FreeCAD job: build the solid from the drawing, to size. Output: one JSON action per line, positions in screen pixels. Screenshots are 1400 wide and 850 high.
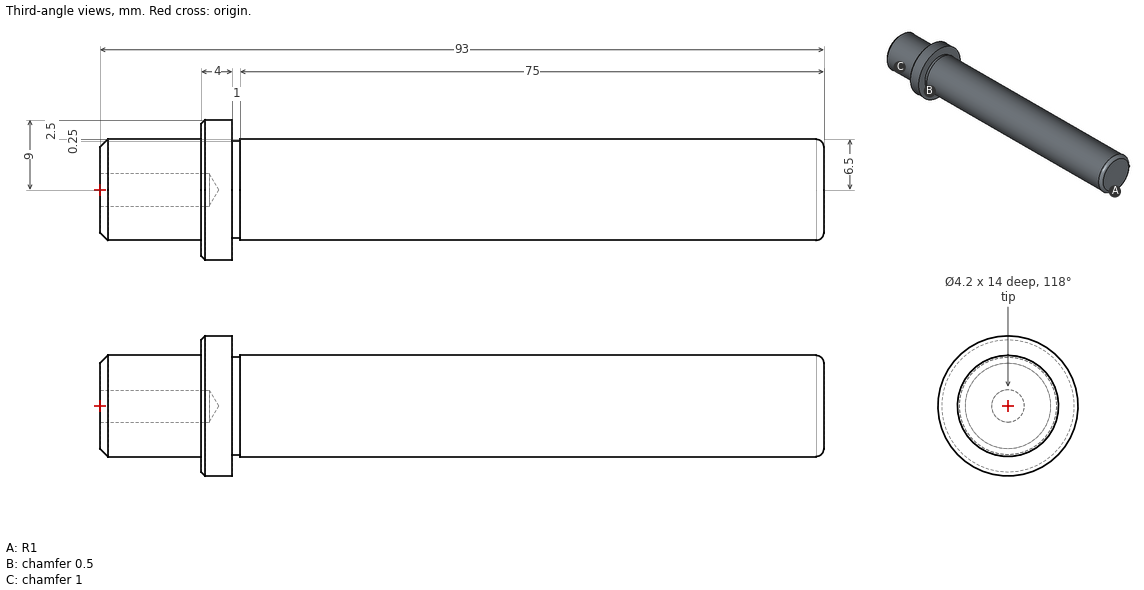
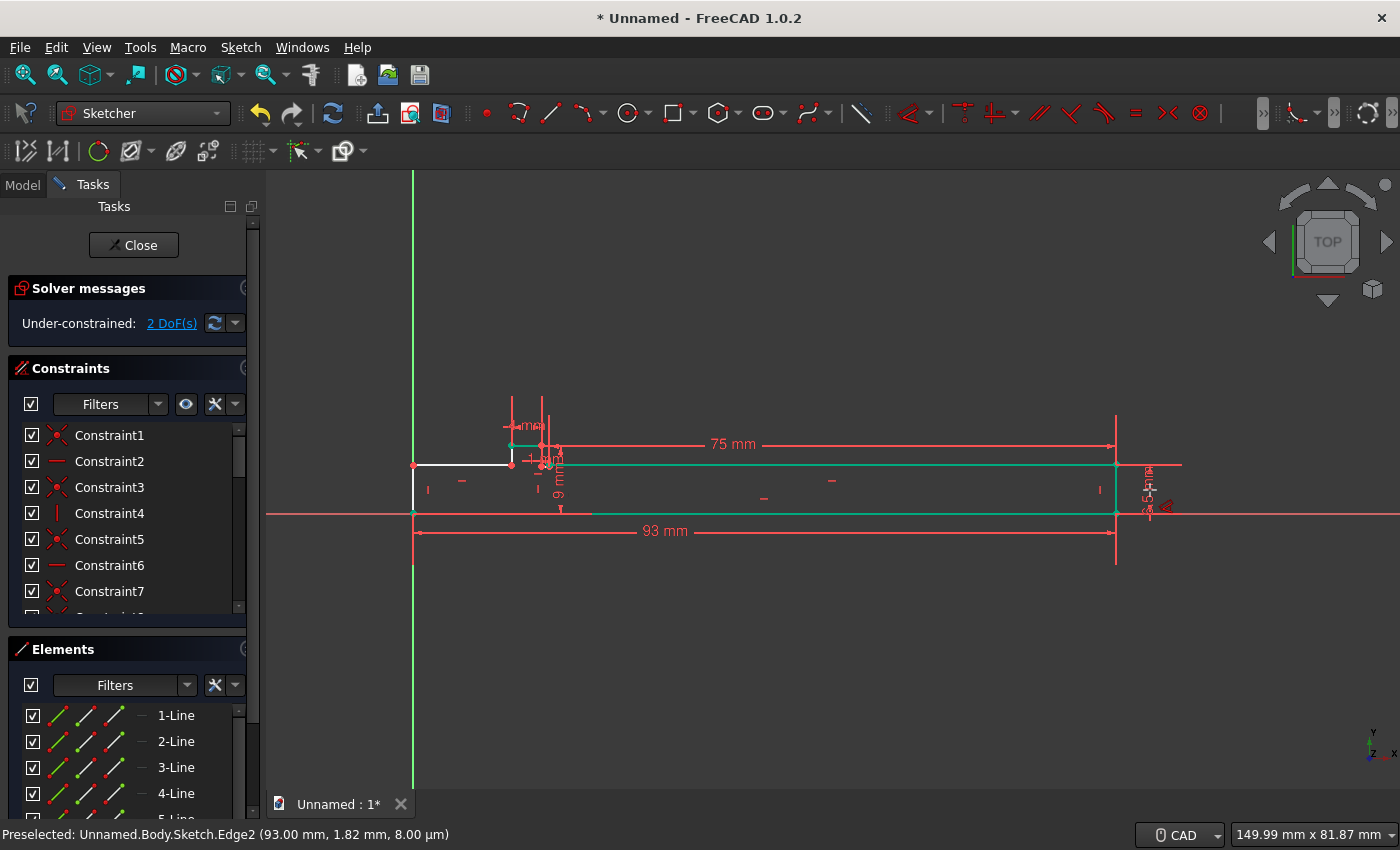
{"action": "scroll", "coordinate": [512, 455], "scroll_direction": "up", "scroll_amount": 4}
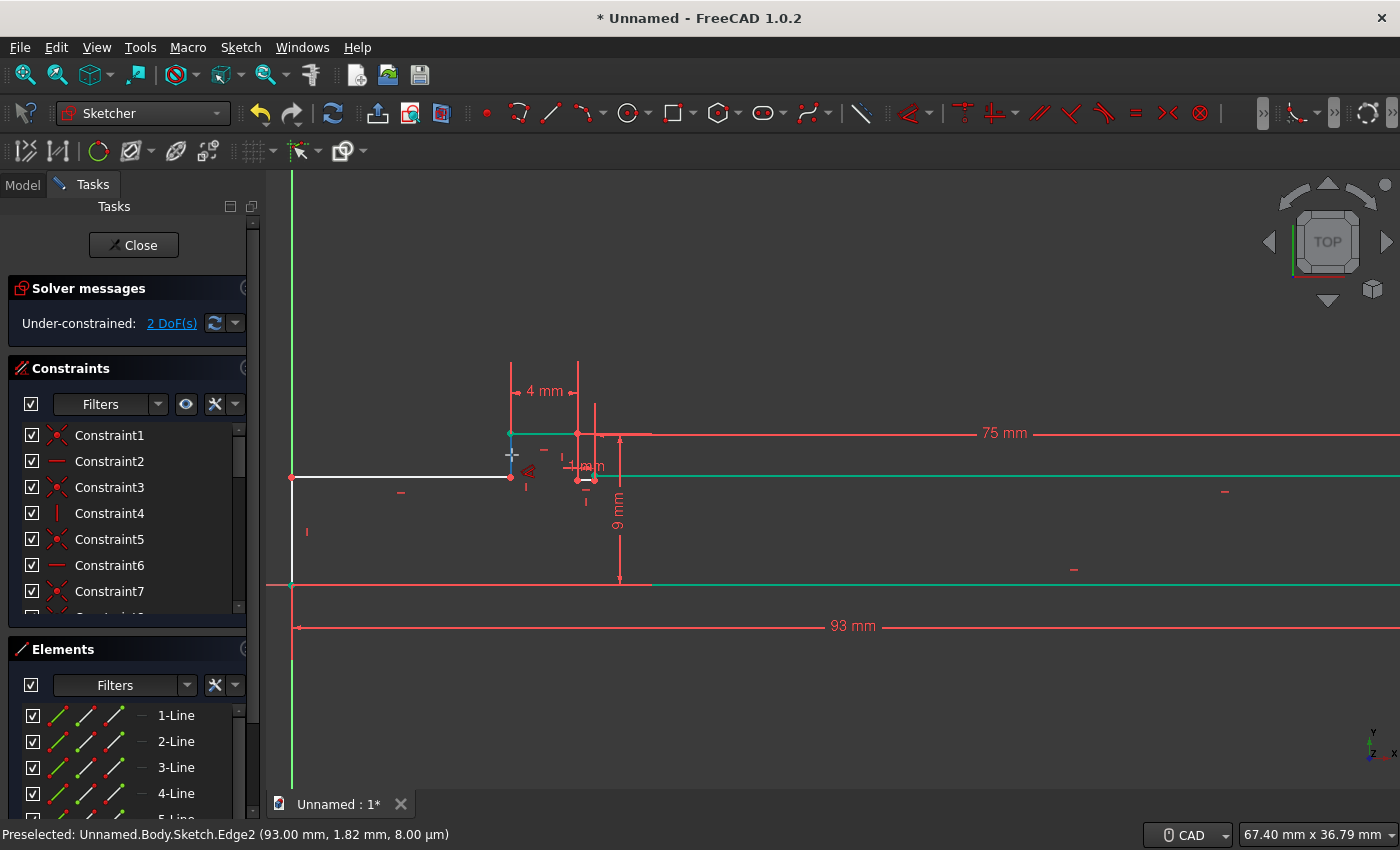
{"action": "left_click", "coordinate": [511, 455]}
{"action": "left_click", "coordinate": [477, 455]}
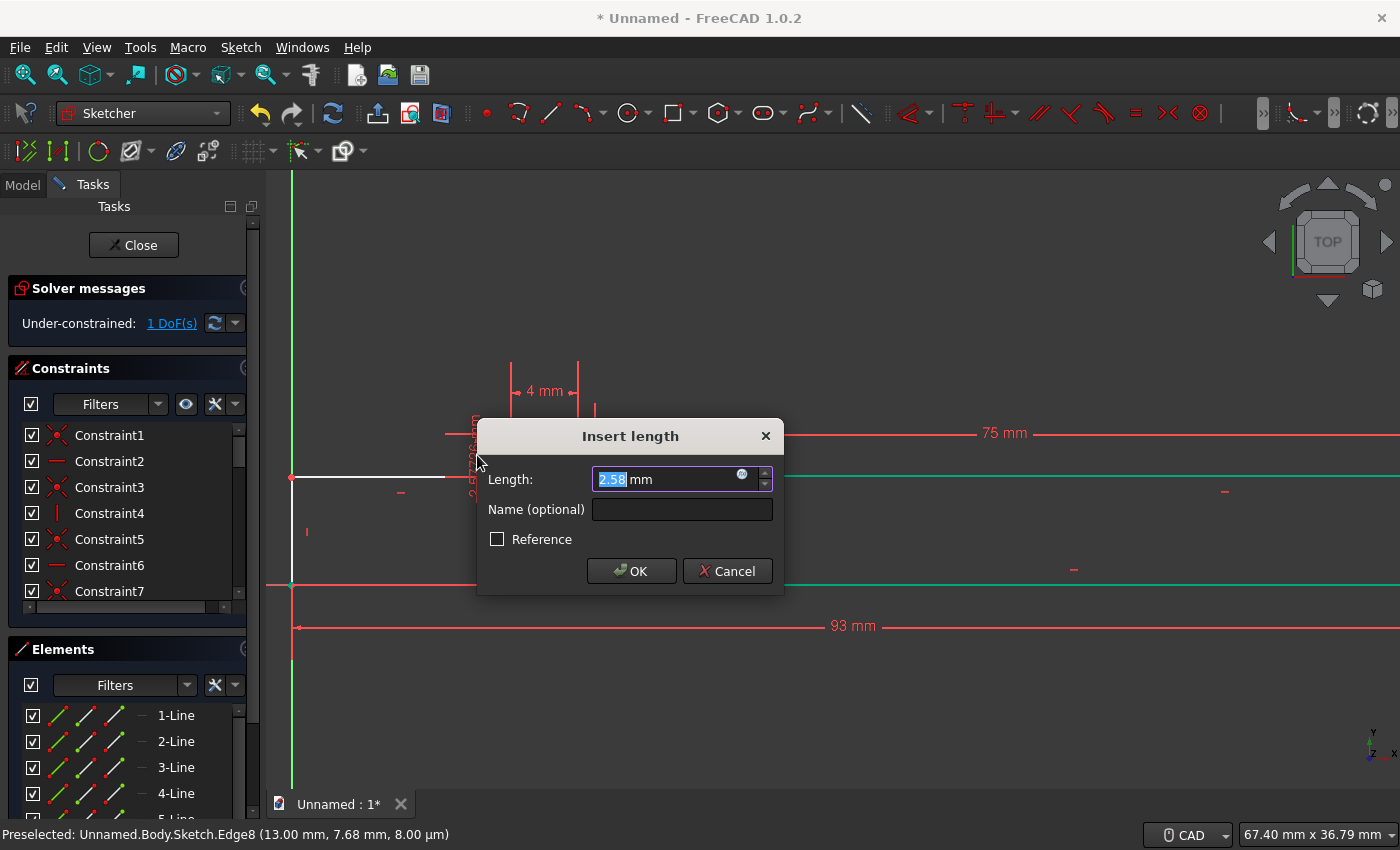
{"action": "type", "text": "2.5"}
{"action": "key", "text": "Return"}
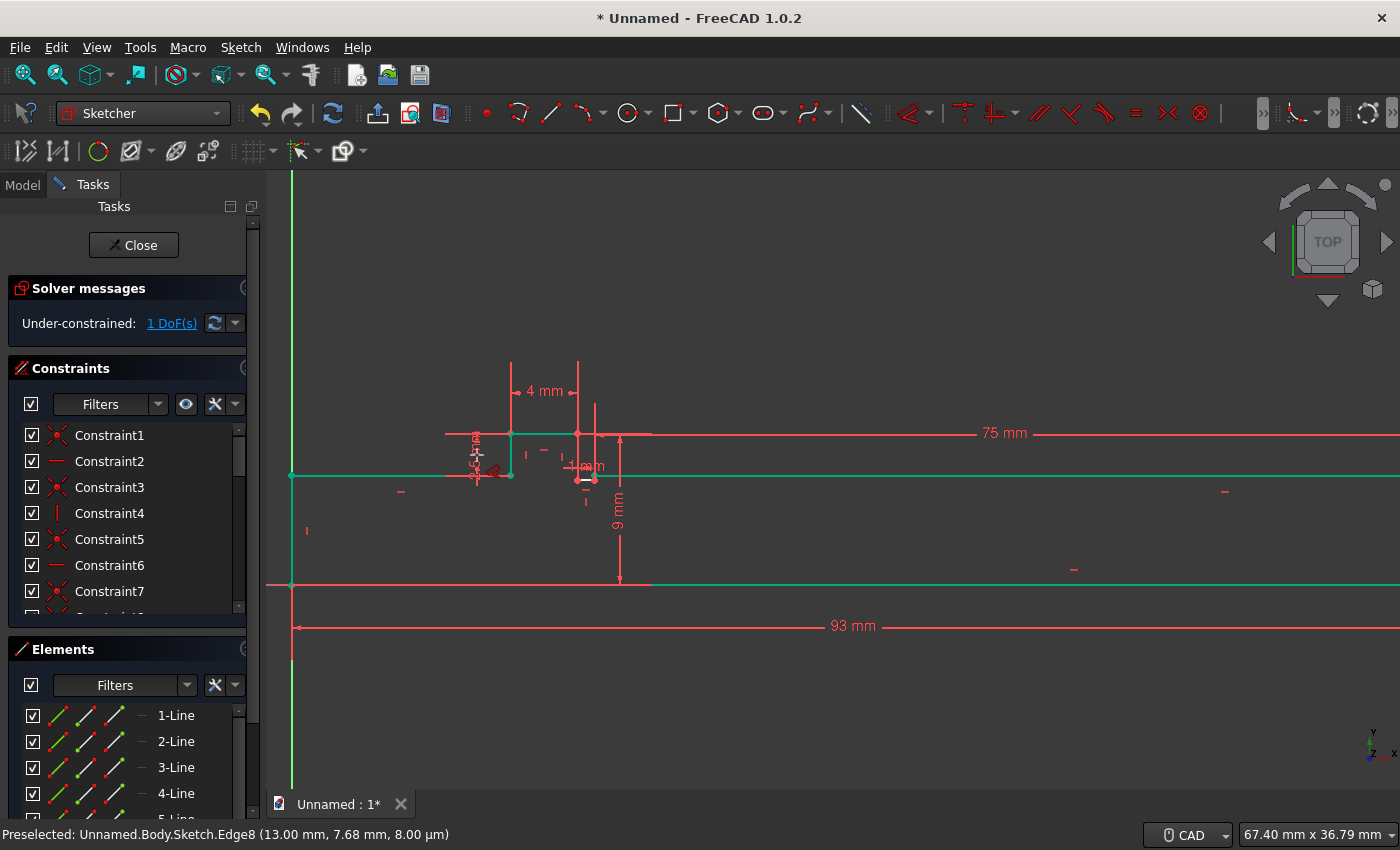
{"action": "scroll", "coordinate": [595, 478], "scroll_direction": "up", "scroll_amount": 12}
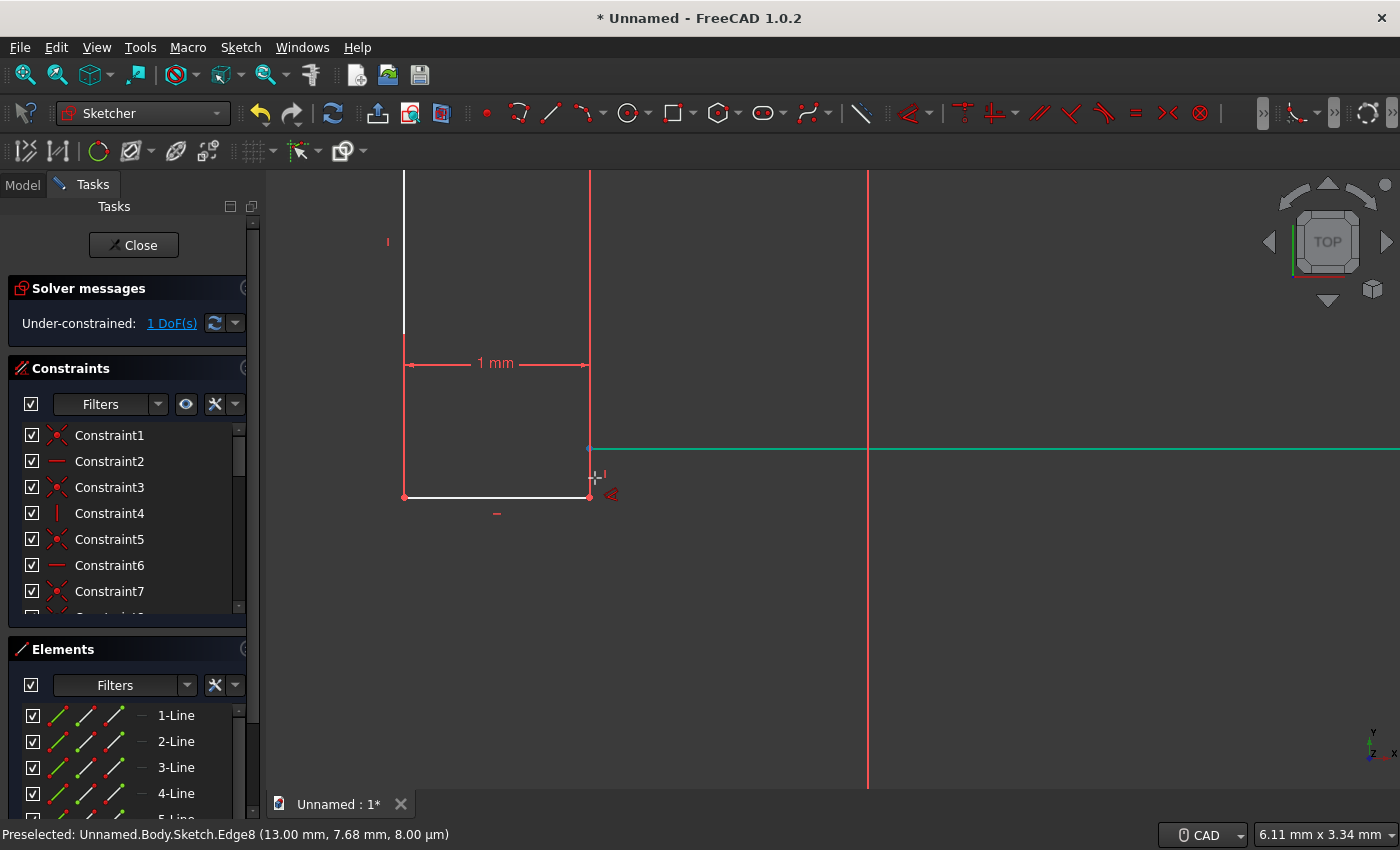
{"action": "left_click", "coordinate": [590, 473]}
{"action": "left_click", "coordinate": [556, 473]}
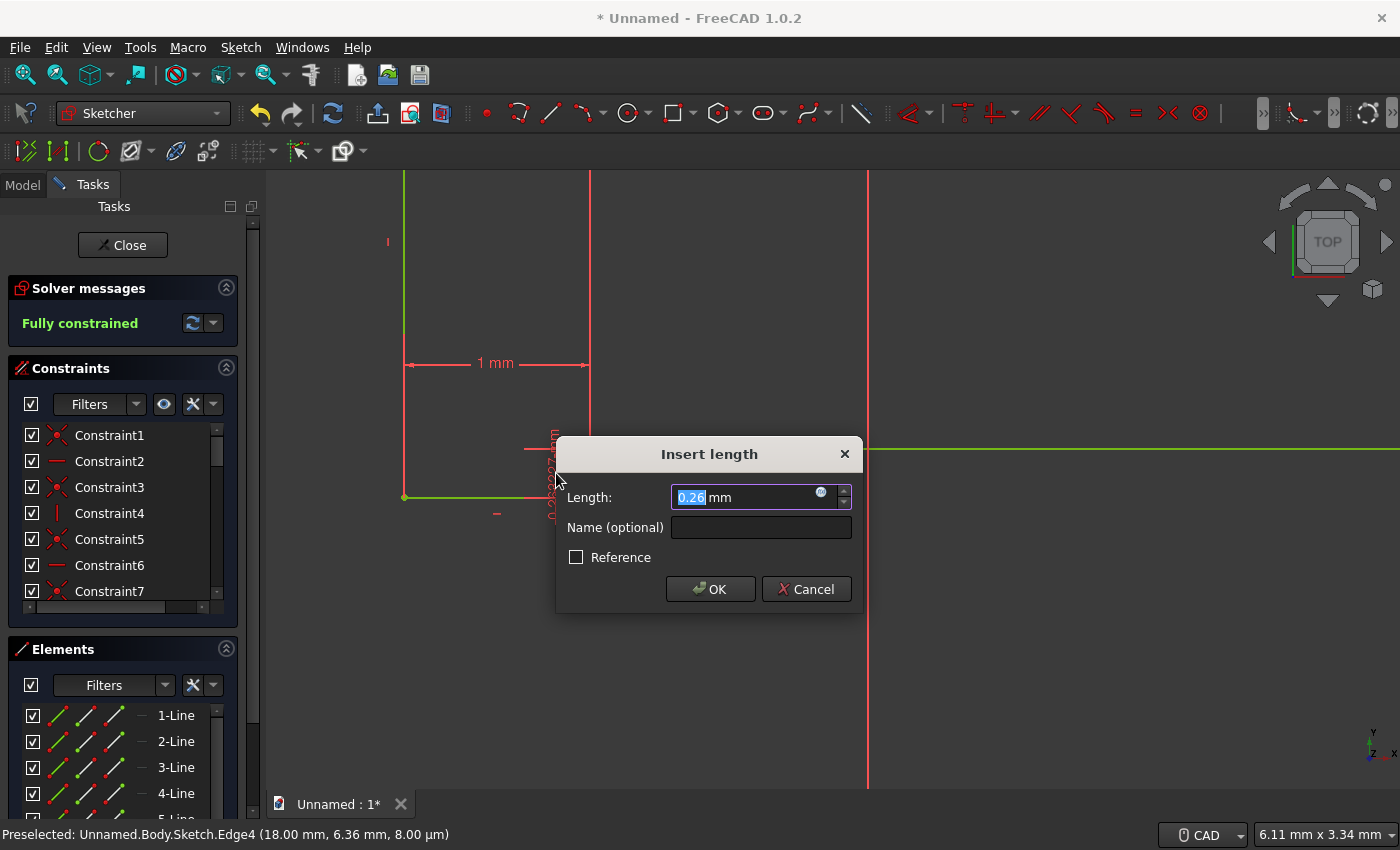
{"action": "type", "text": "0.25"}
{"action": "key", "text": "Return"}
{"action": "key", "text": "Escape"}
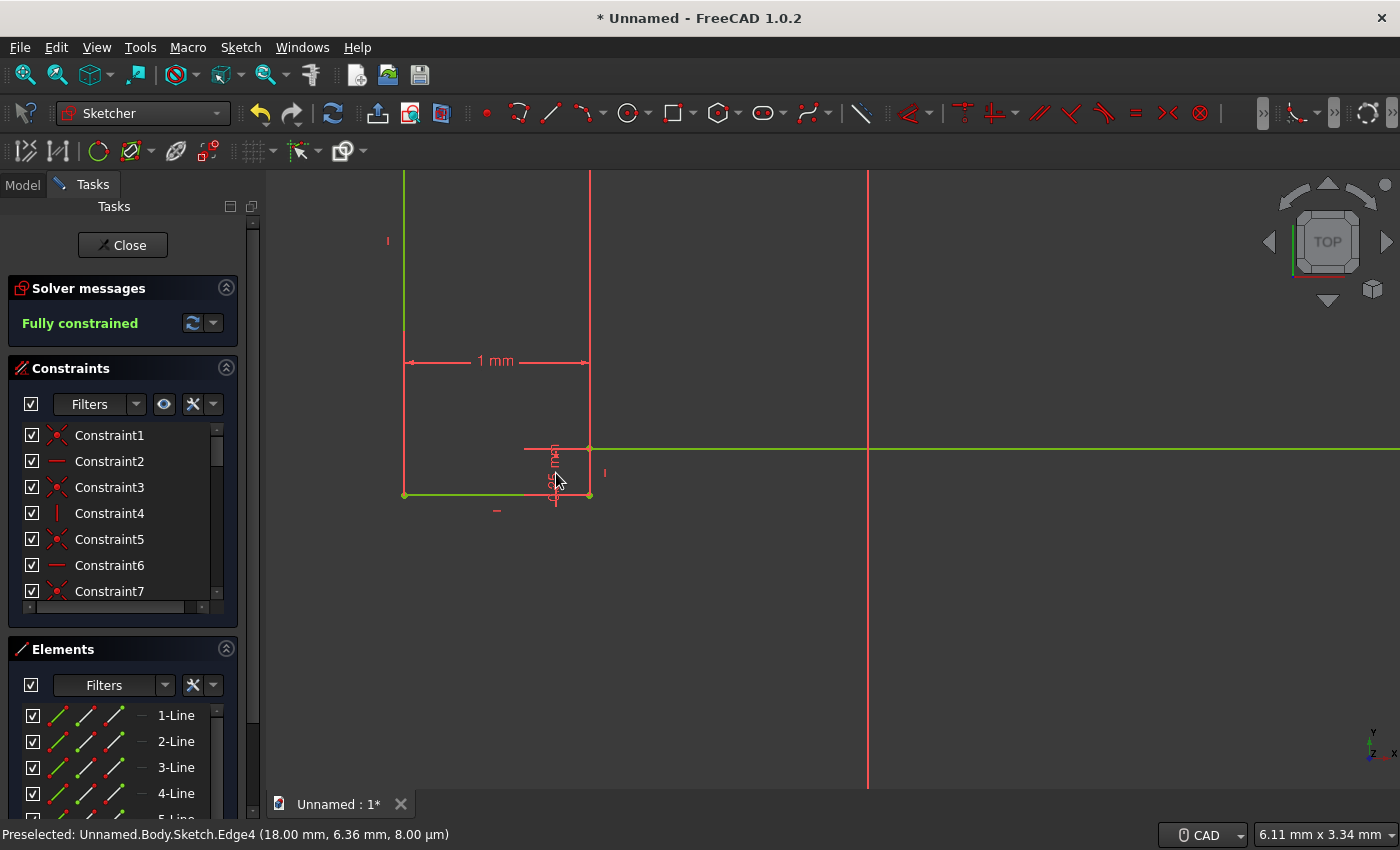
{"action": "left_click", "coordinate": [123, 245]}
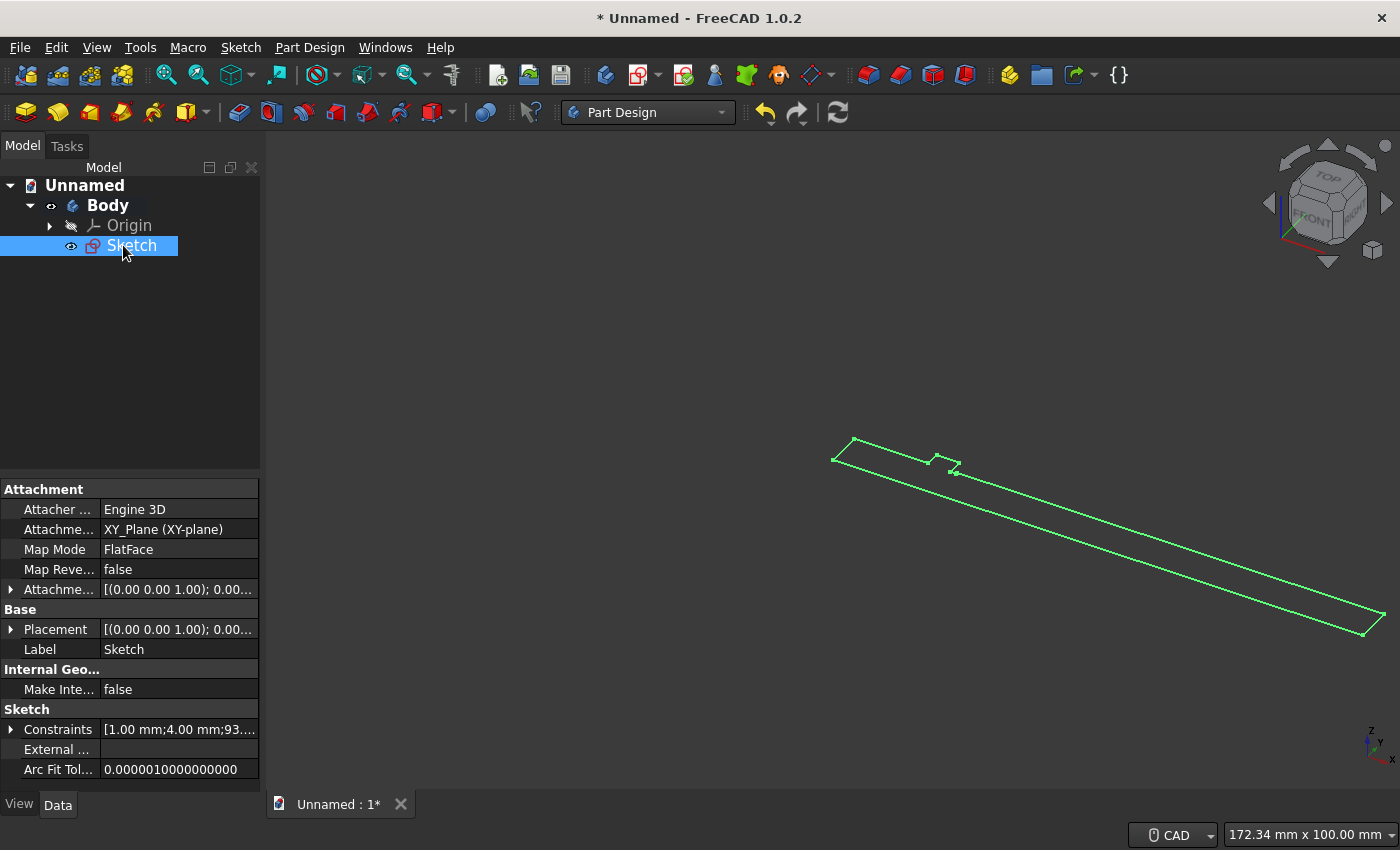
{"action": "left_click", "coordinate": [58, 112]}